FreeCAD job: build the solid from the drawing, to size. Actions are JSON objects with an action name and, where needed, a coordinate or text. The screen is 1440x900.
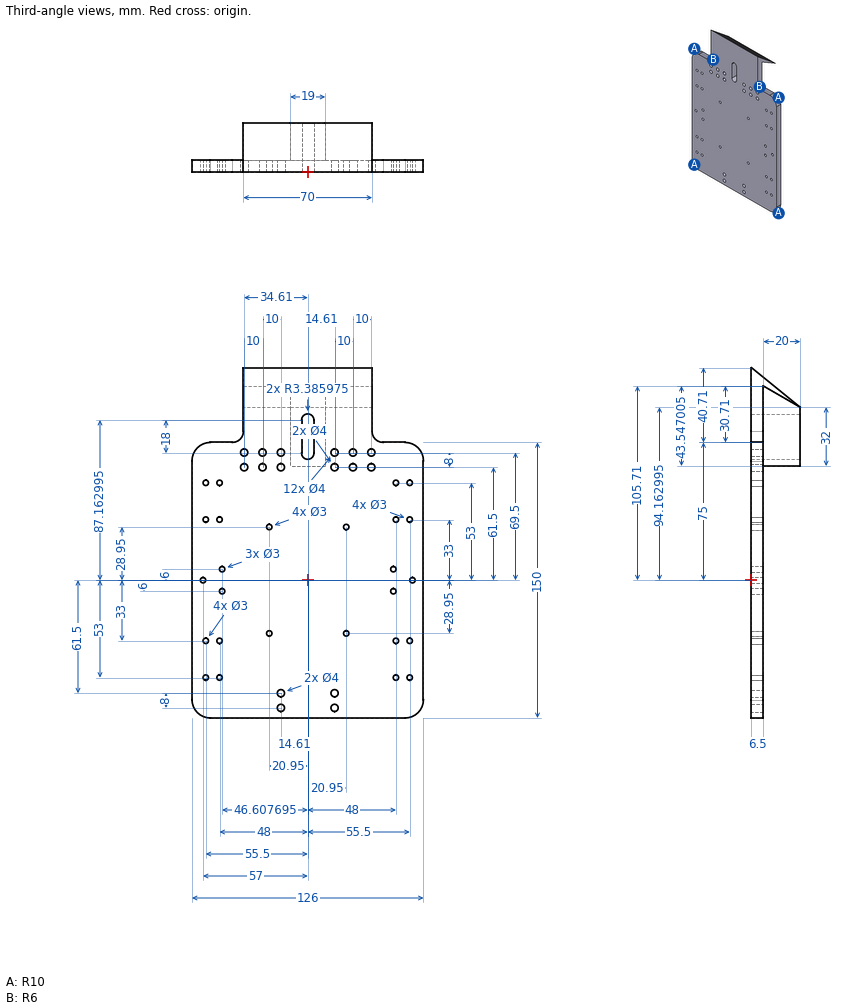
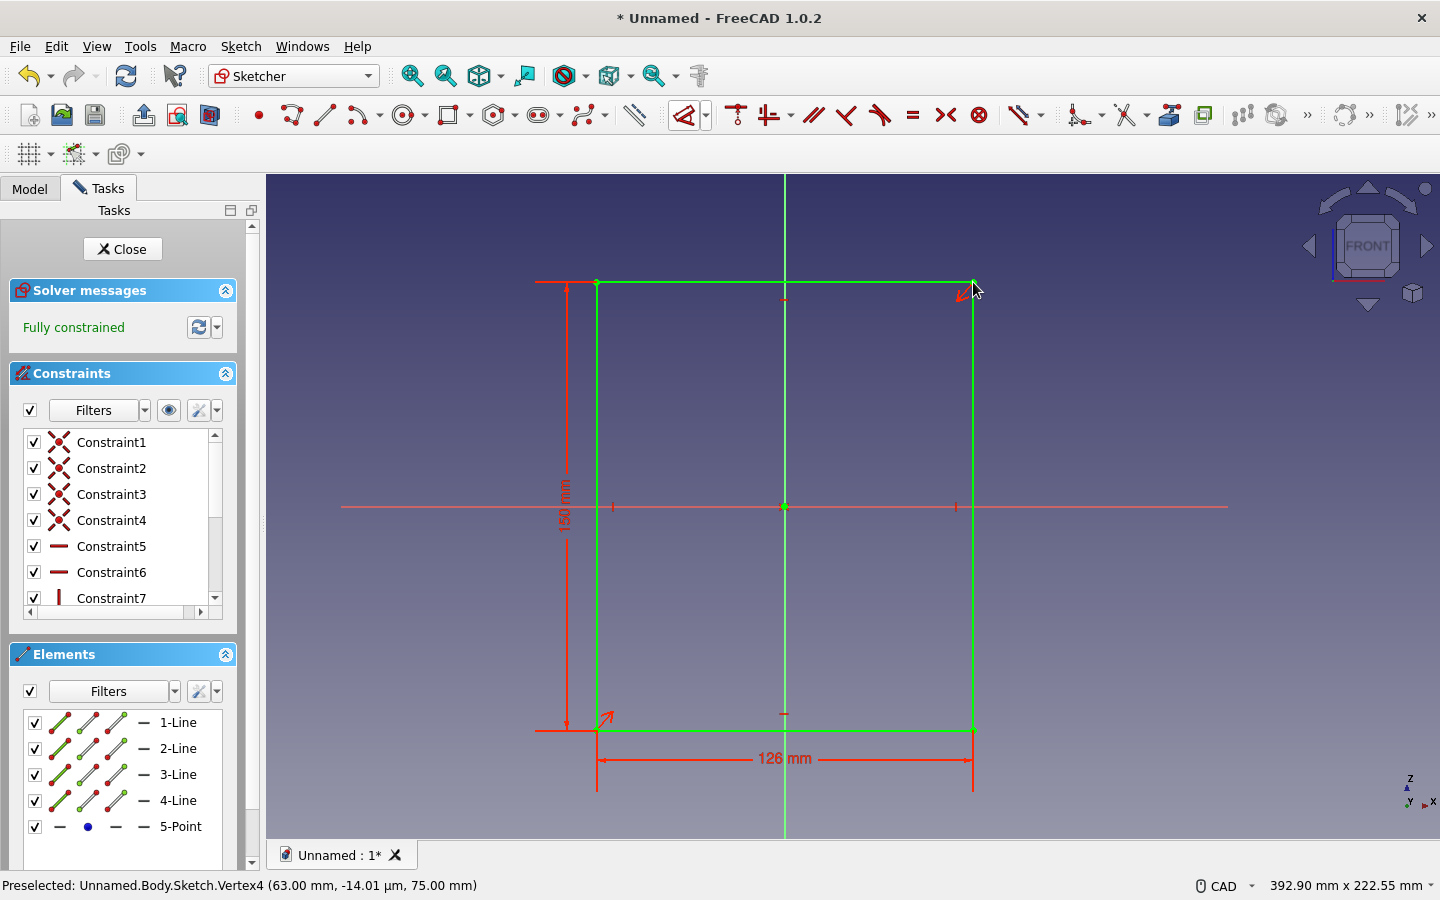
{"action": "left_click", "coordinate": [123, 249]}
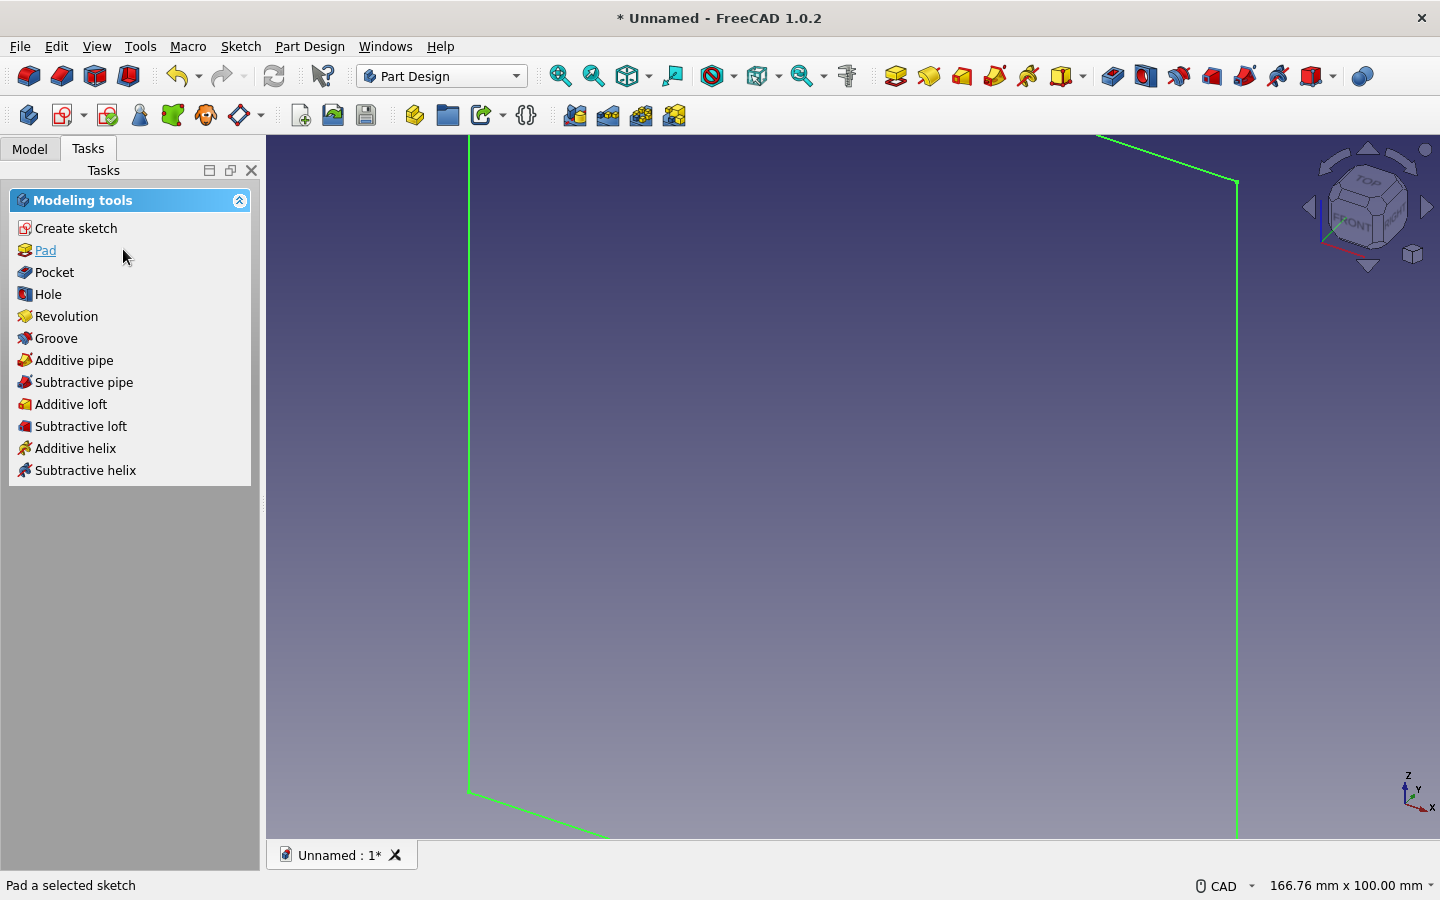
{"action": "left_click", "coordinate": [896, 76]}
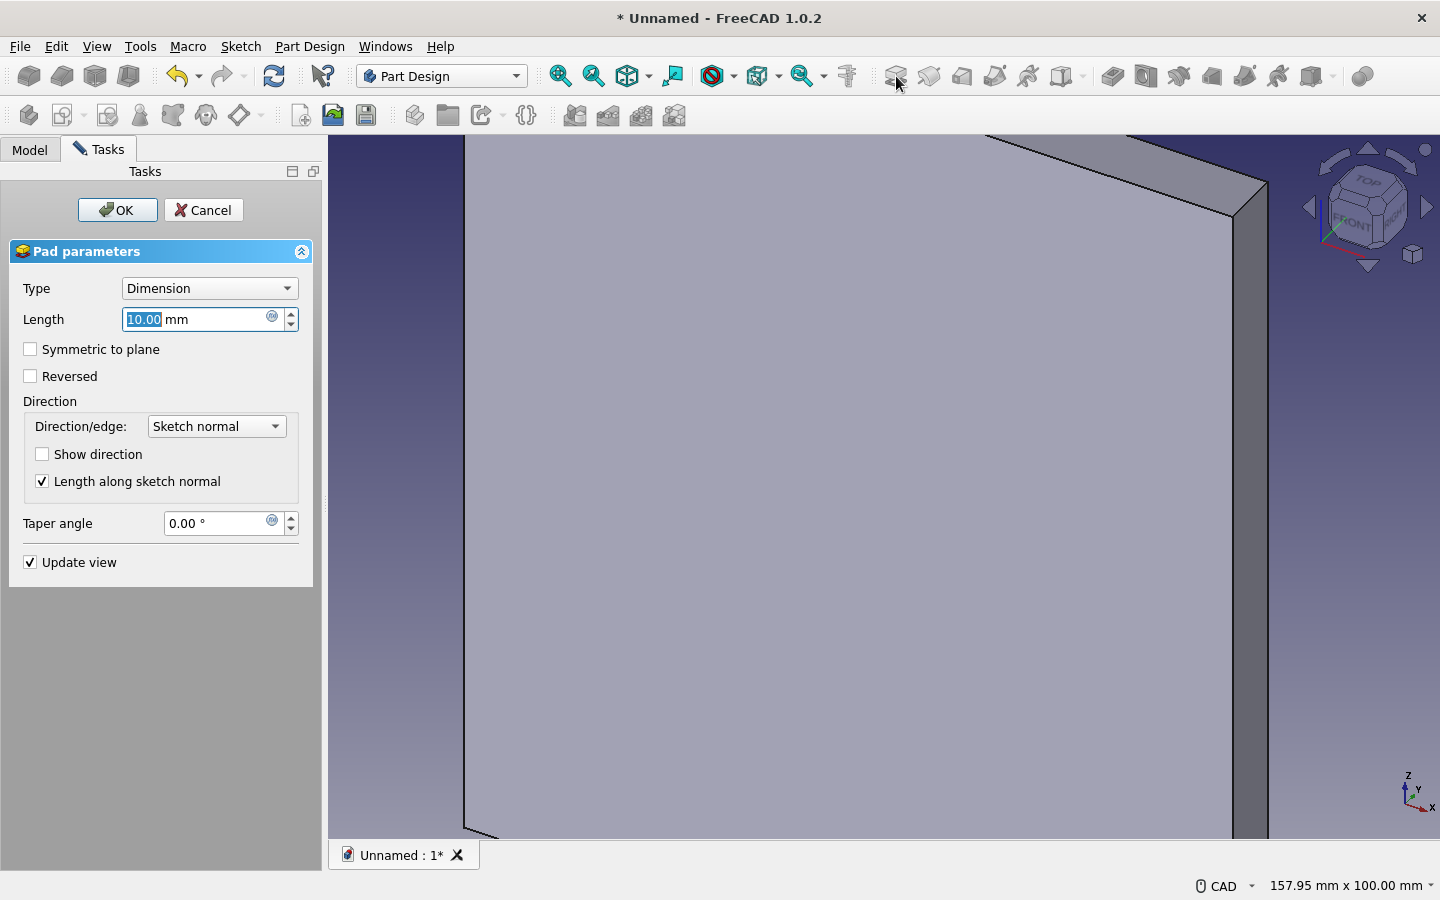
{"action": "type", "text": "6.5"}
{"action": "key", "text": "Tab"}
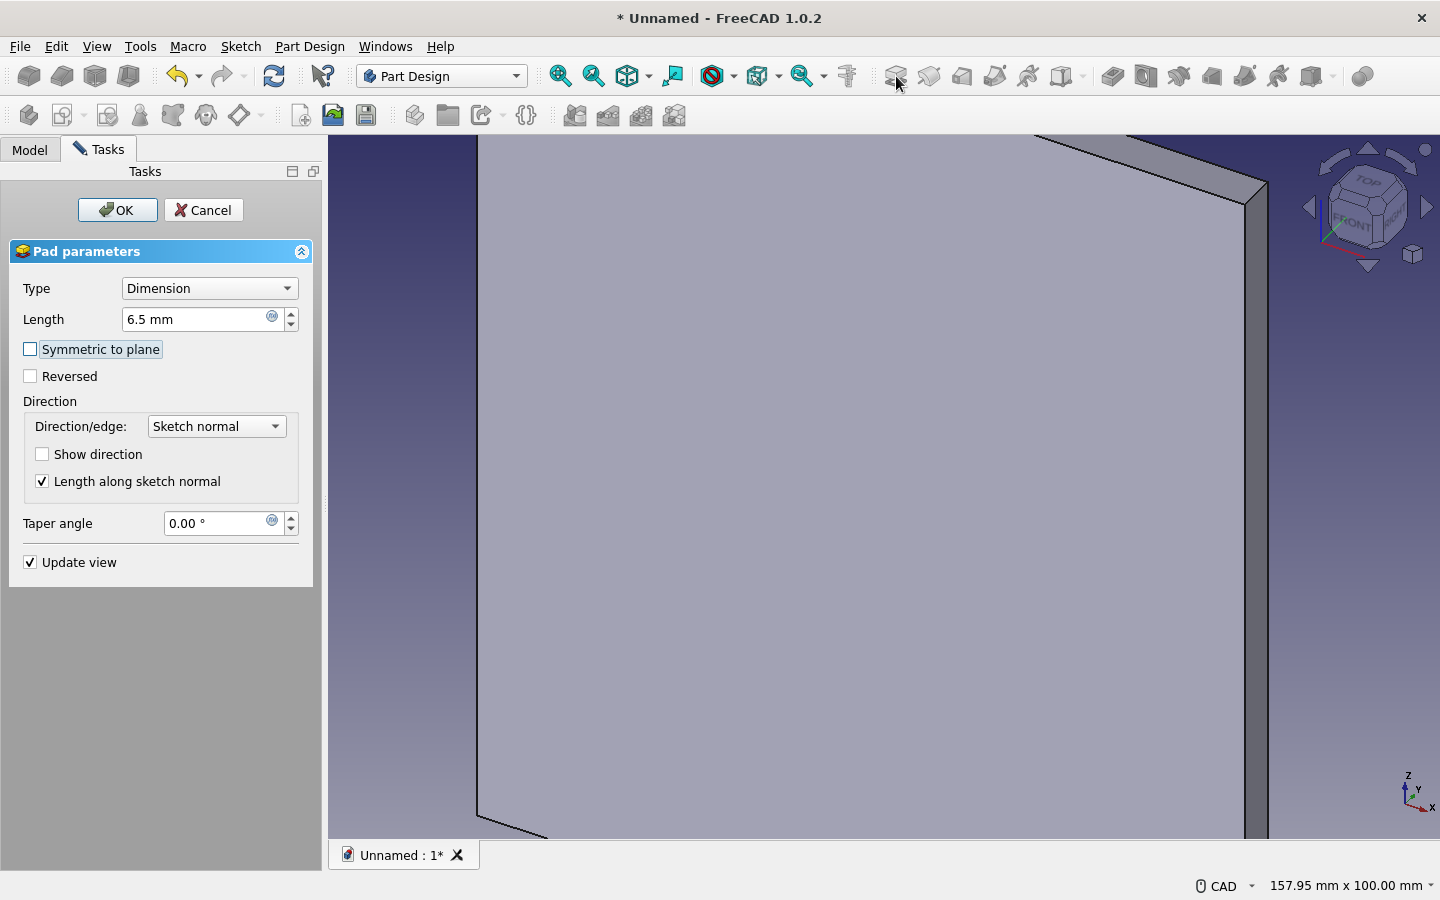
{"action": "left_click", "coordinate": [31, 376]}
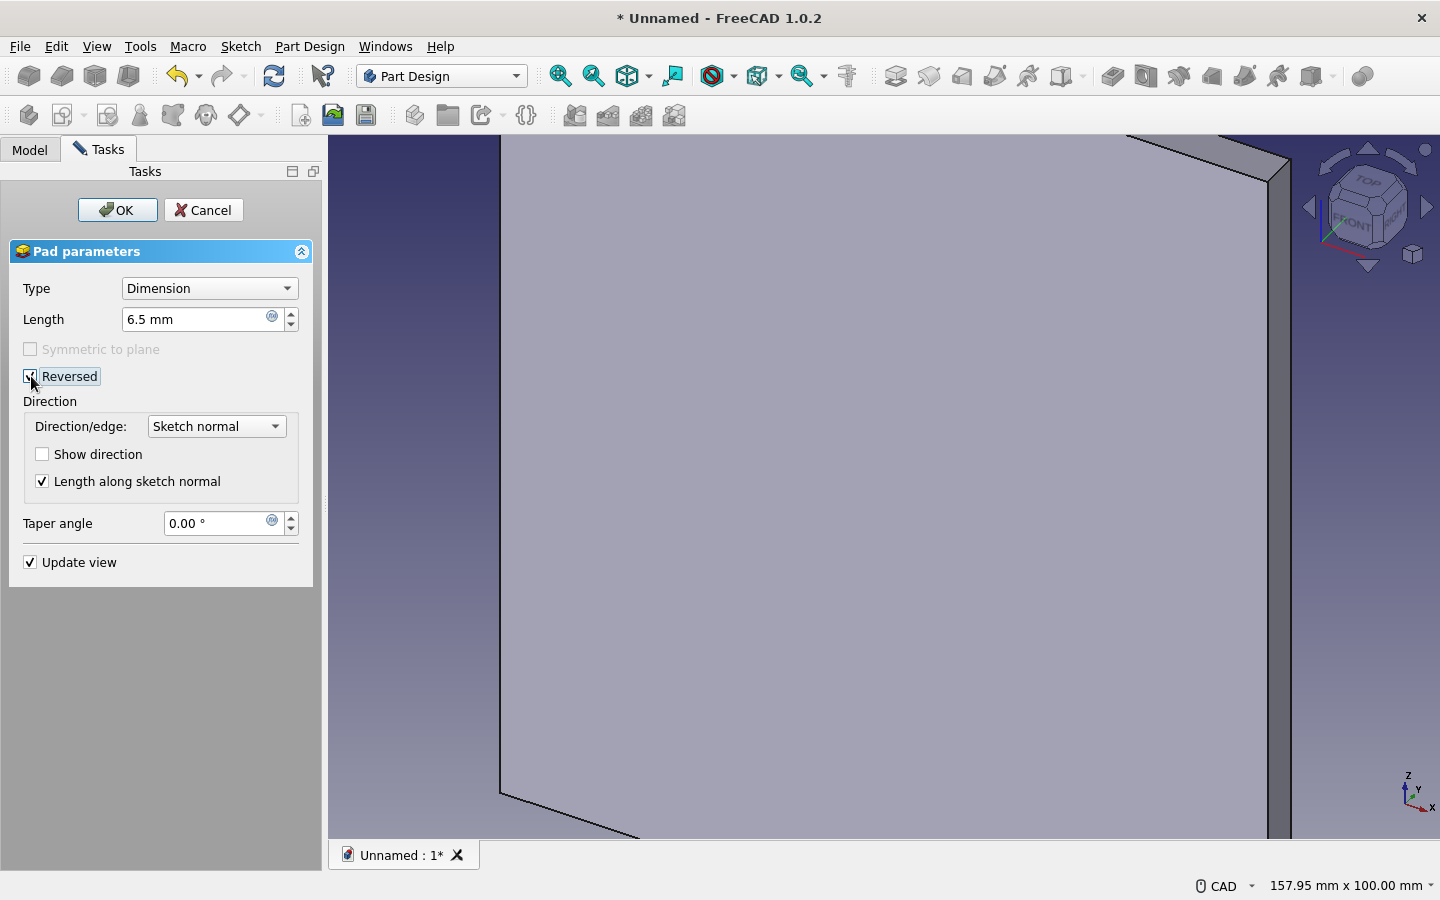
{"action": "left_click", "coordinate": [118, 210]}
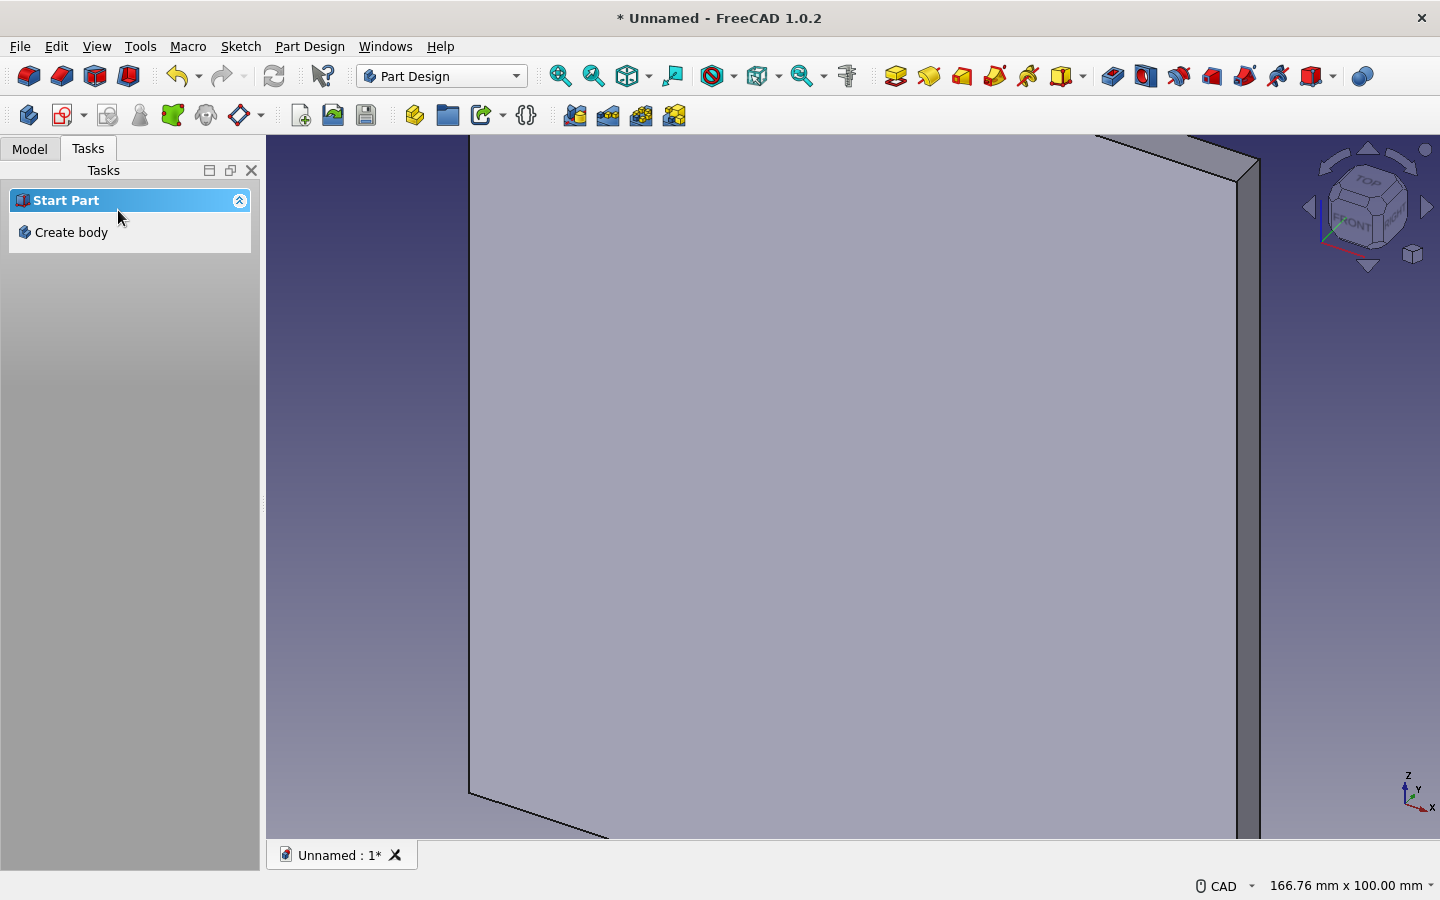
{"action": "left_click", "coordinate": [561, 76]}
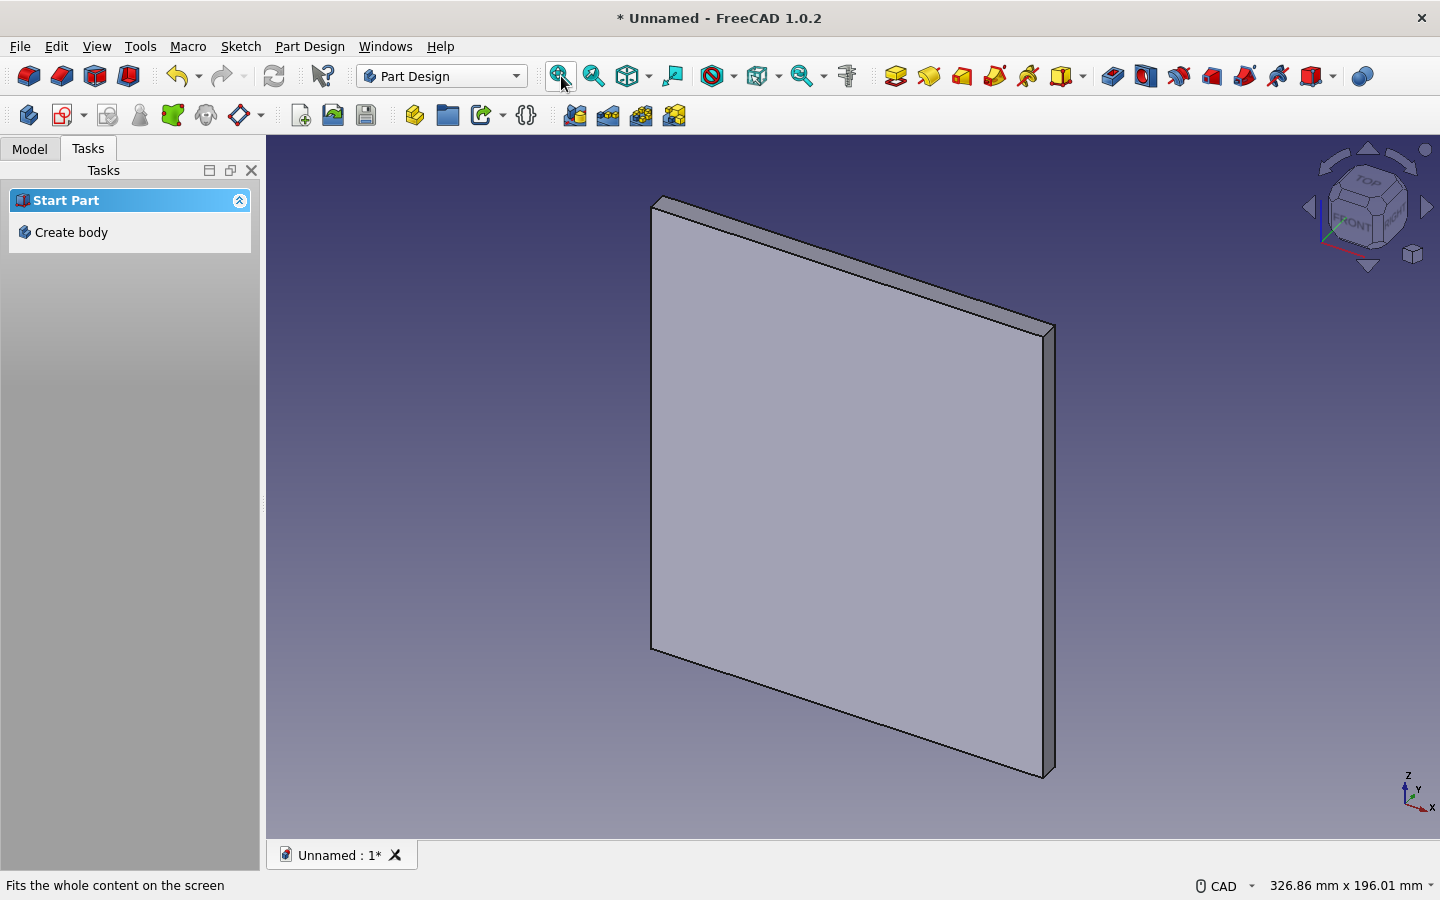
{"action": "key", "text": "4"}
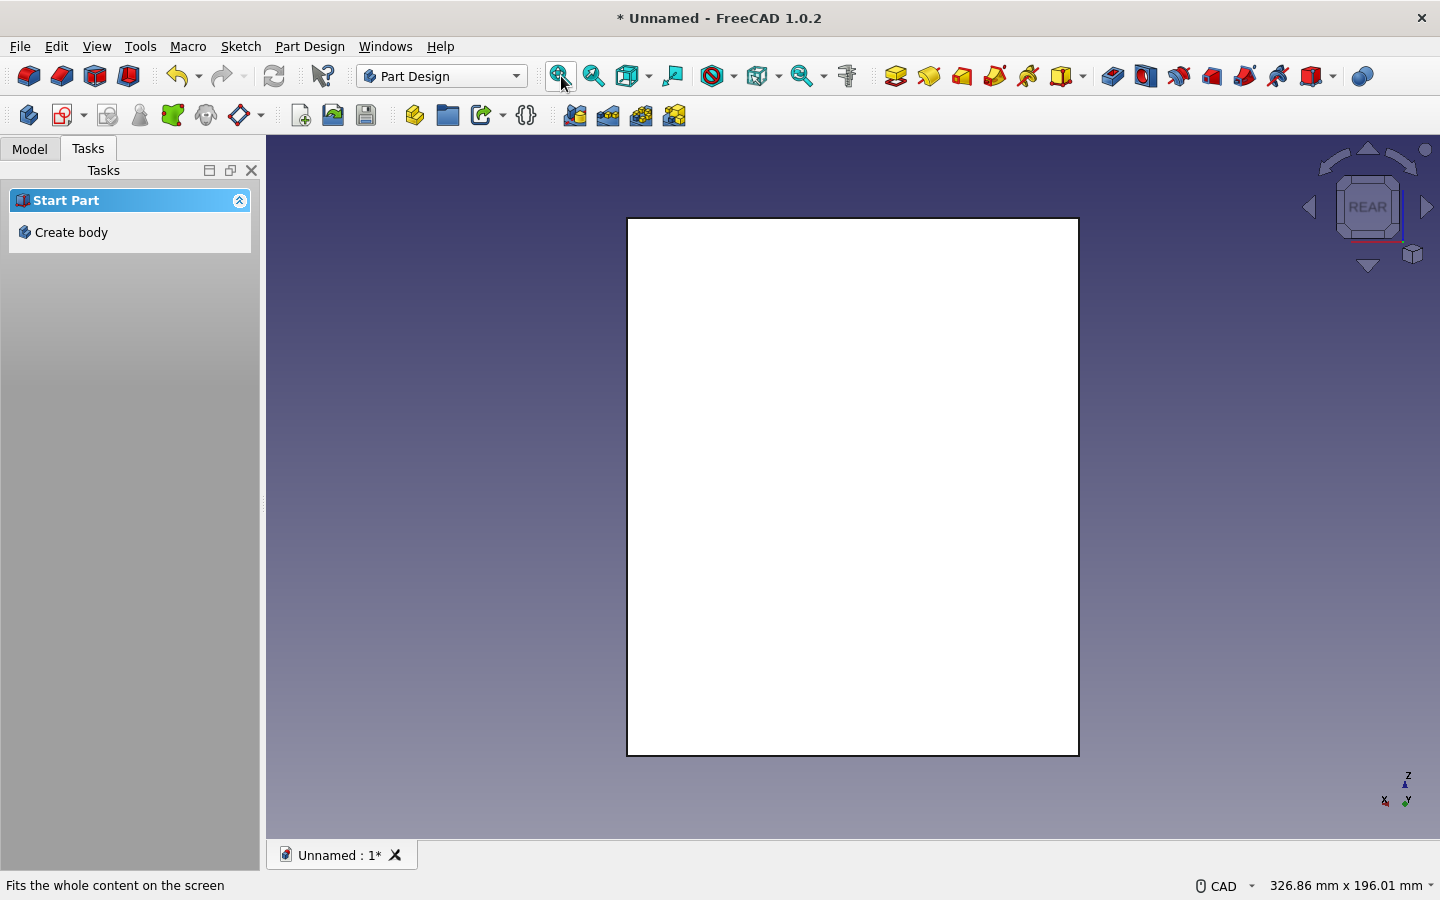
{"action": "left_click", "coordinate": [853, 486]}